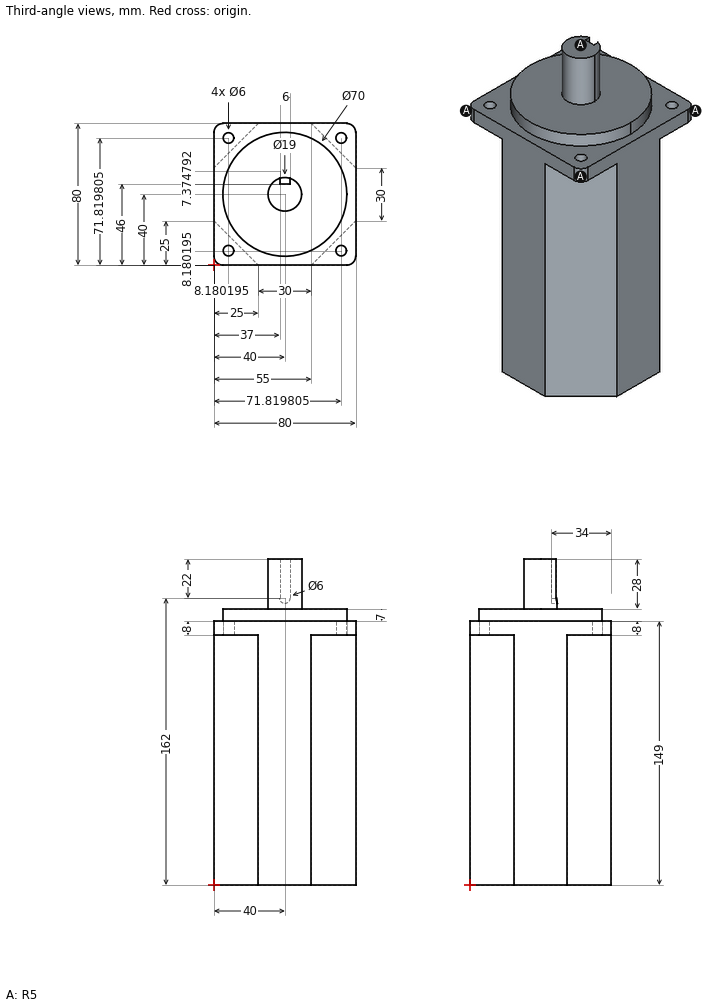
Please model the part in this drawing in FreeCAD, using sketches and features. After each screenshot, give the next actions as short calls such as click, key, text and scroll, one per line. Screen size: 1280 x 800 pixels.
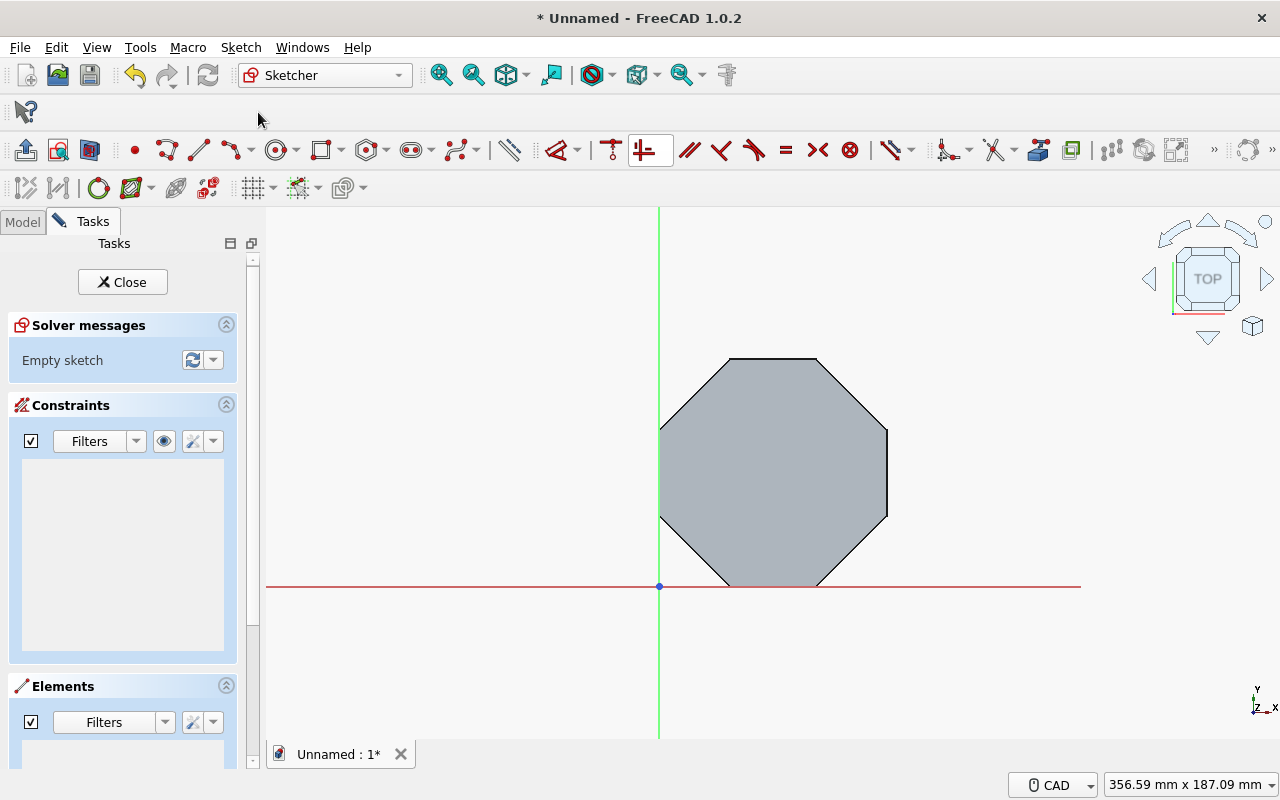
scroll(891, 495, up, 2)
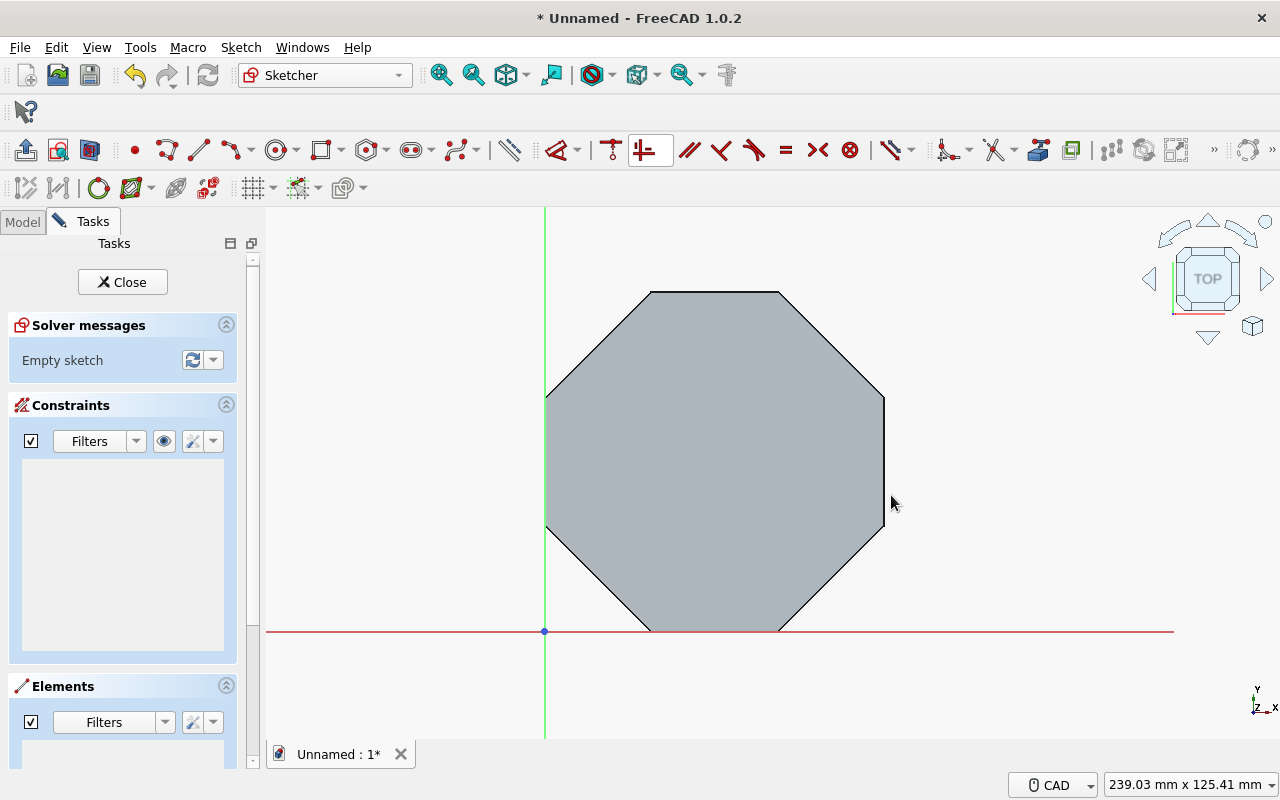
click(276, 150)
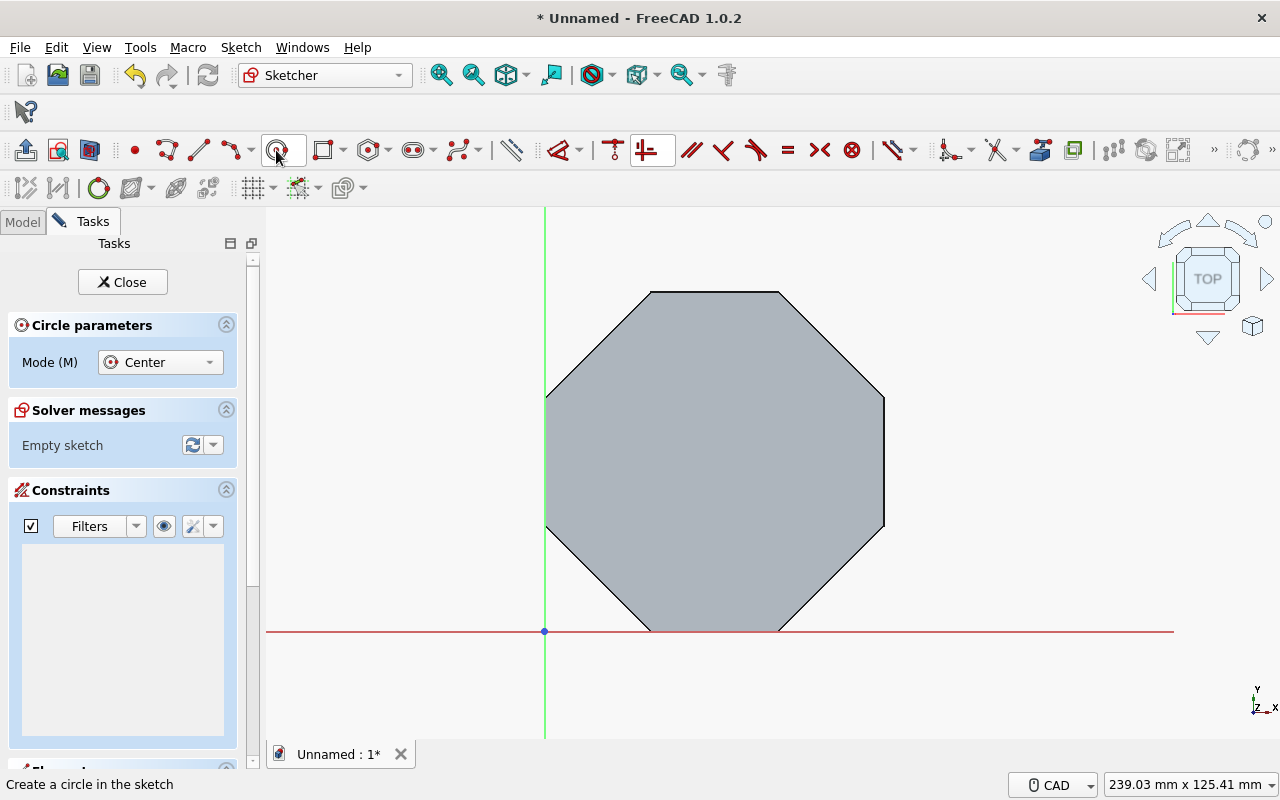
click(715, 462)
click(820, 357)
key(Escape)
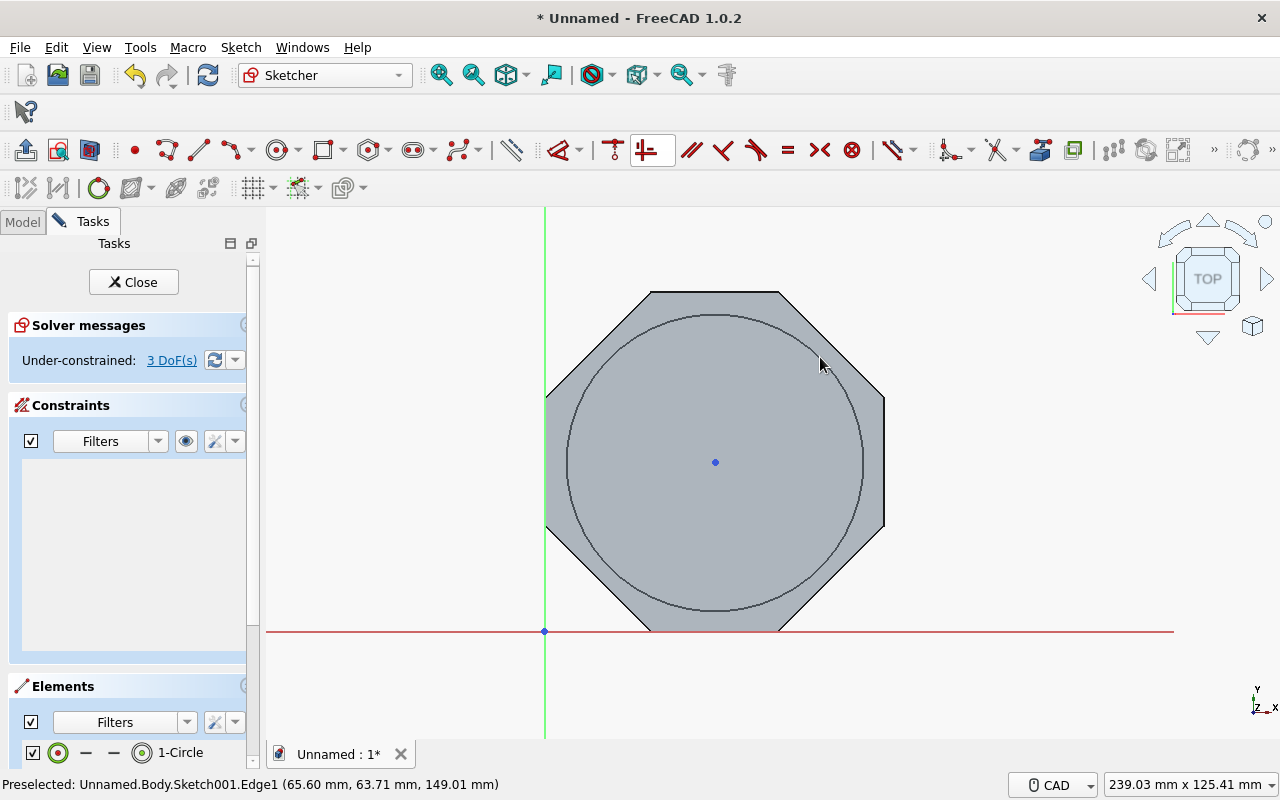
key(d)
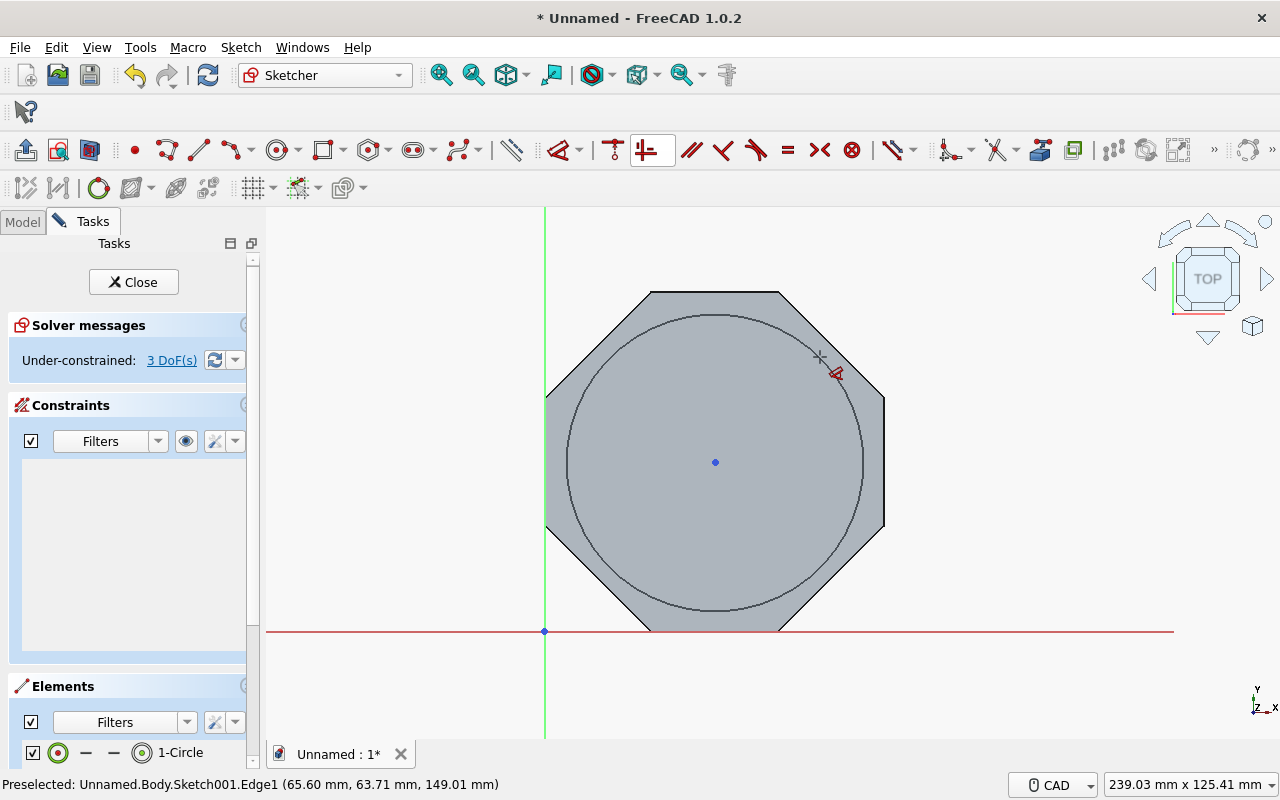
click(820, 358)
click(843, 335)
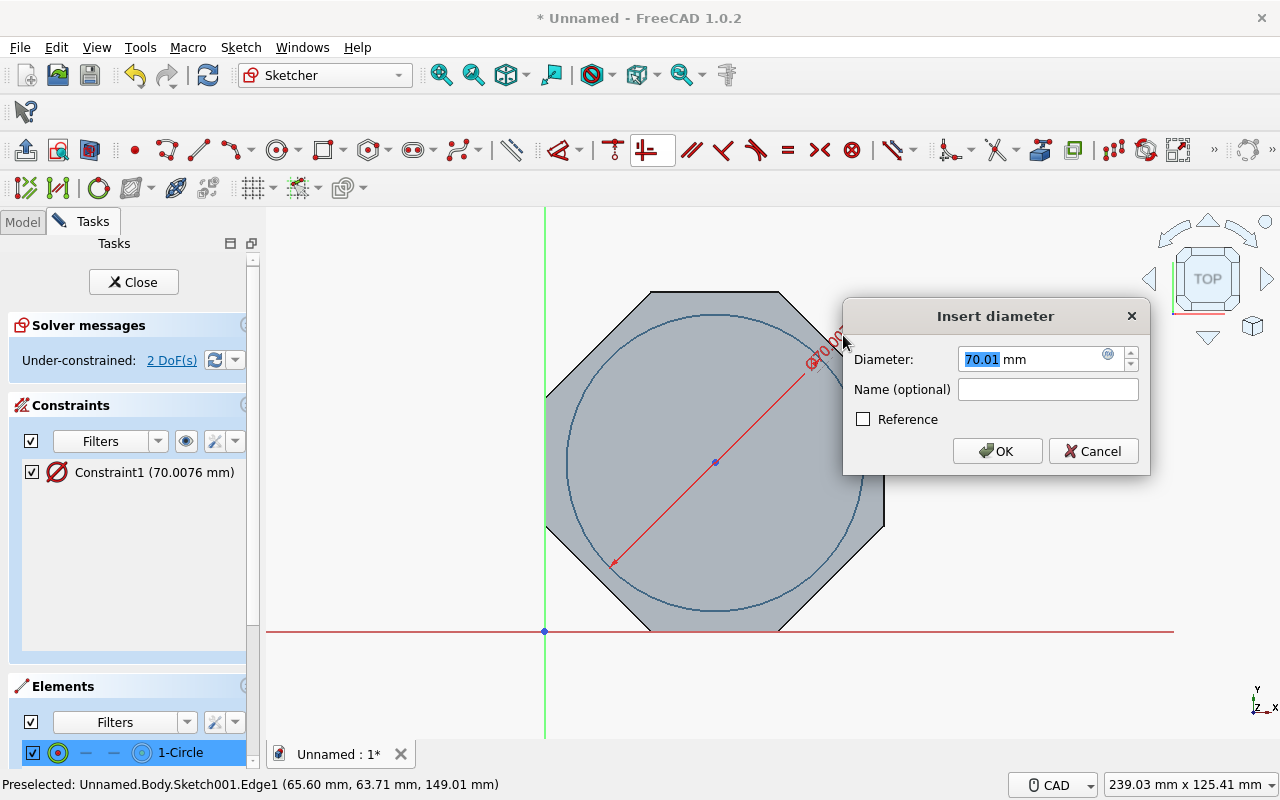
text(70)
key(Return)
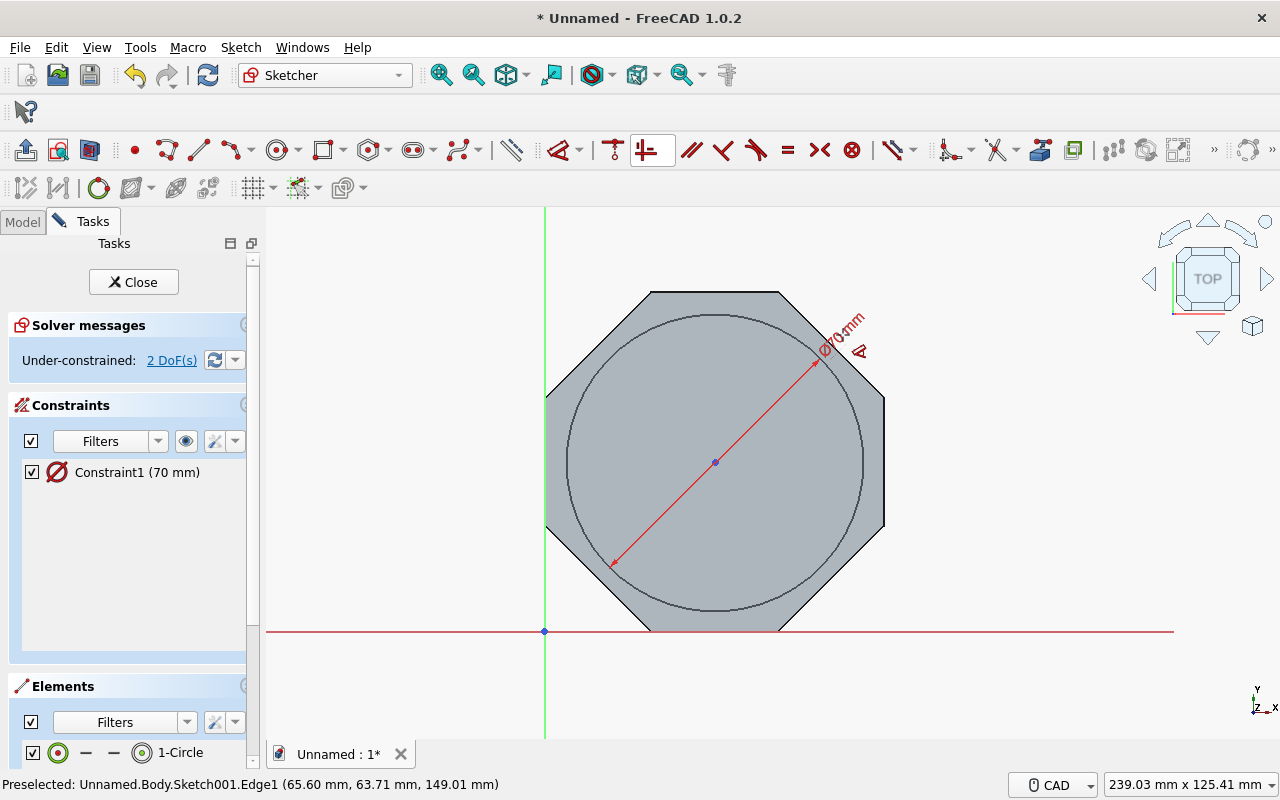
click(715, 463)
click(630, 666)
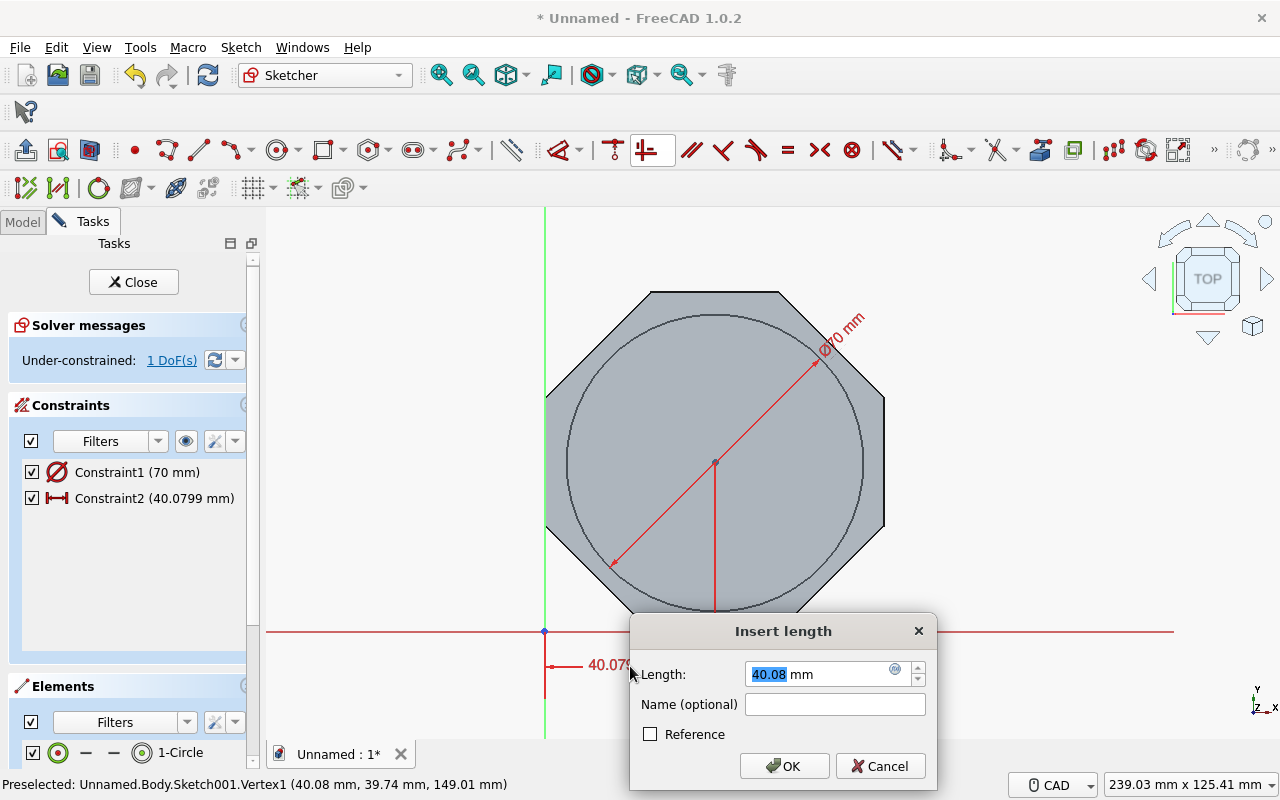
text(40)
key(Return)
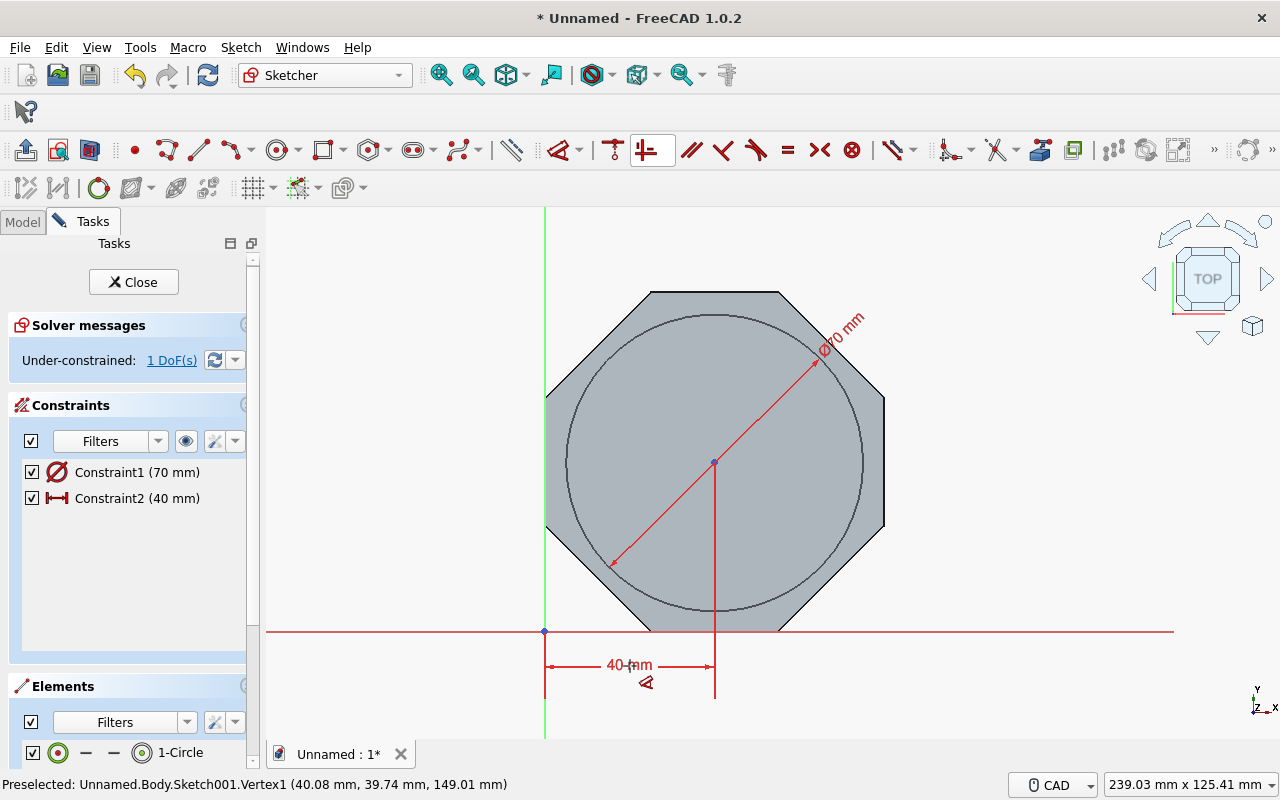
click(715, 463)
click(511, 547)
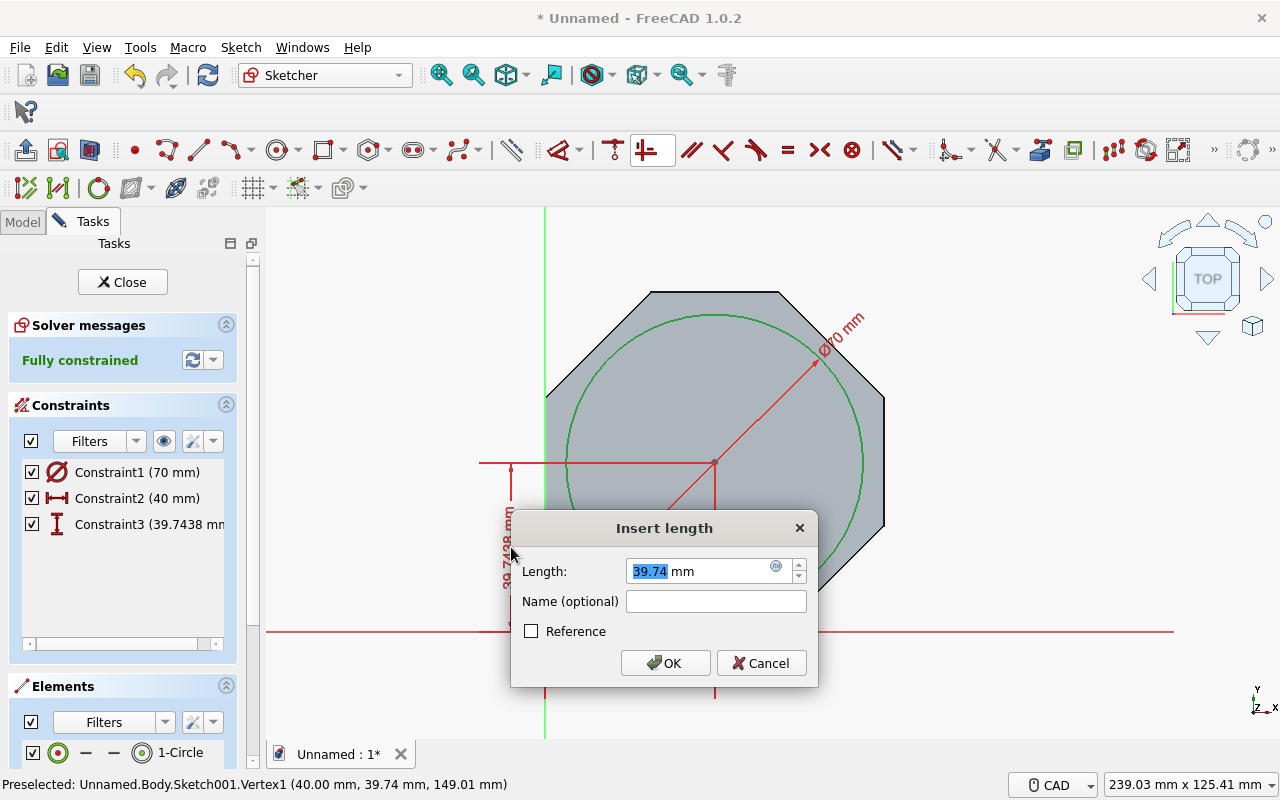
text(40)
key(Return)
key(Escape)